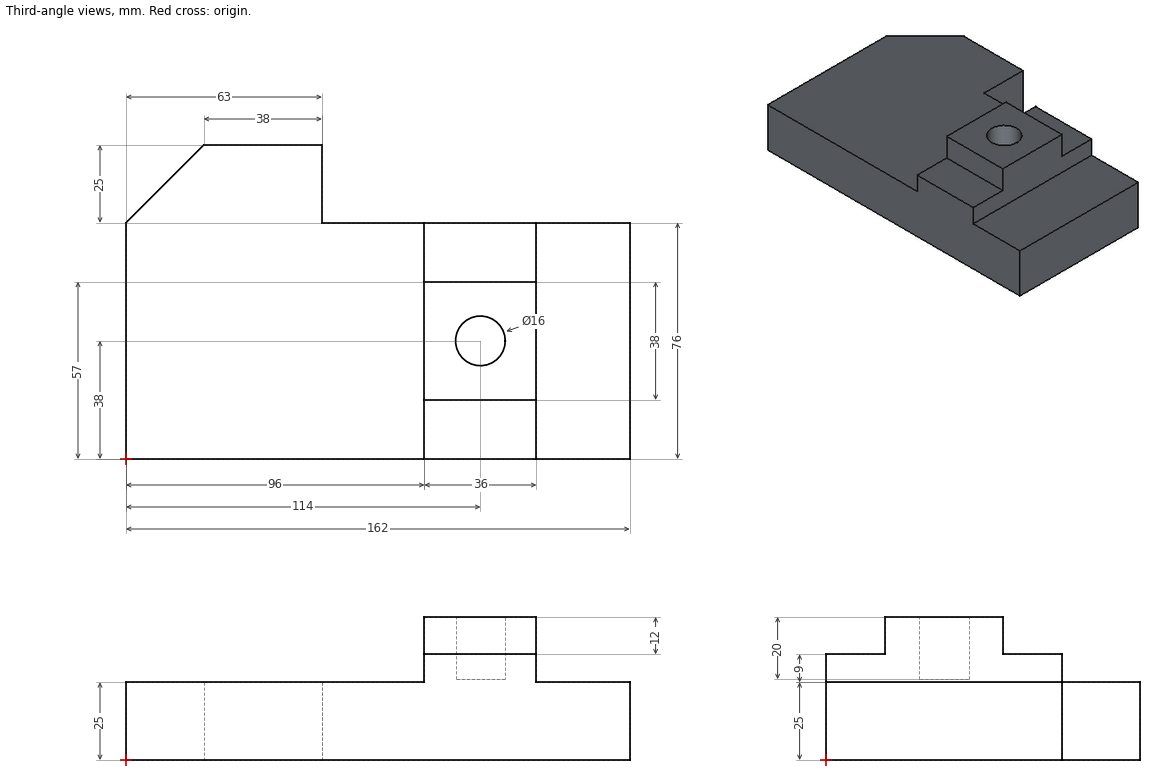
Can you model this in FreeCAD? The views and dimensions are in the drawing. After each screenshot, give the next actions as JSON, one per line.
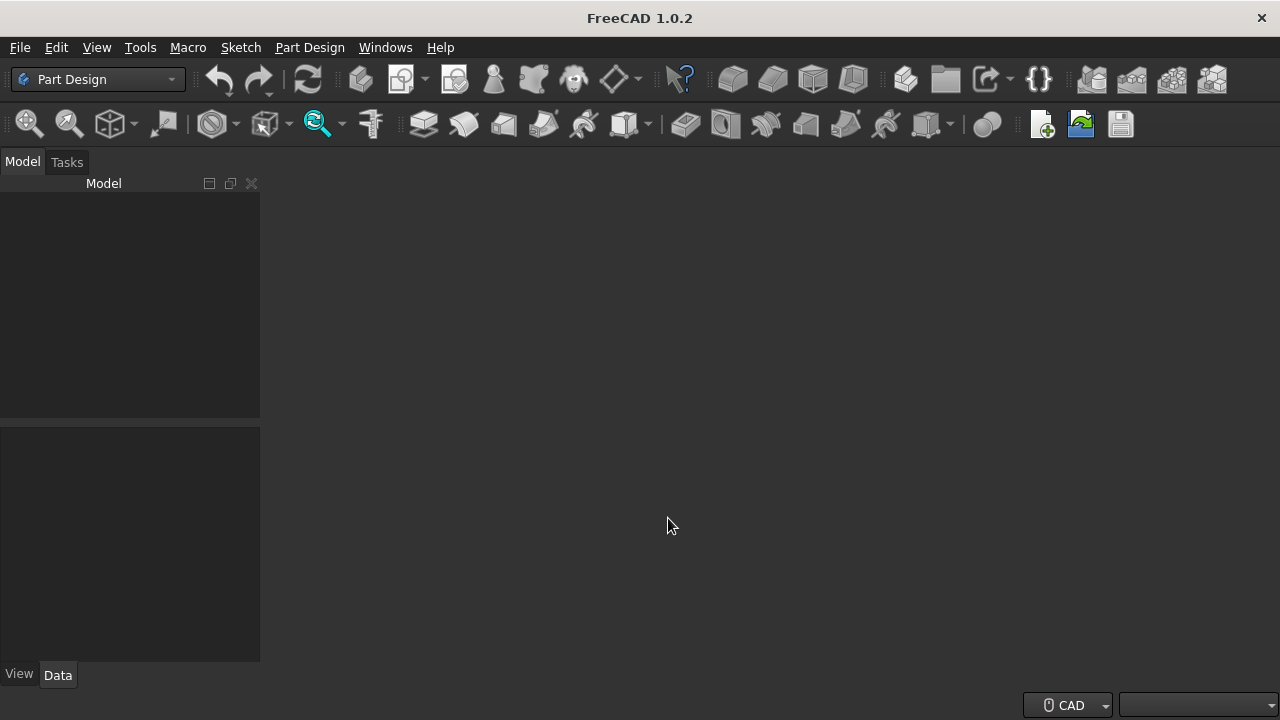
{"action": "key", "text": "ctrl+n"}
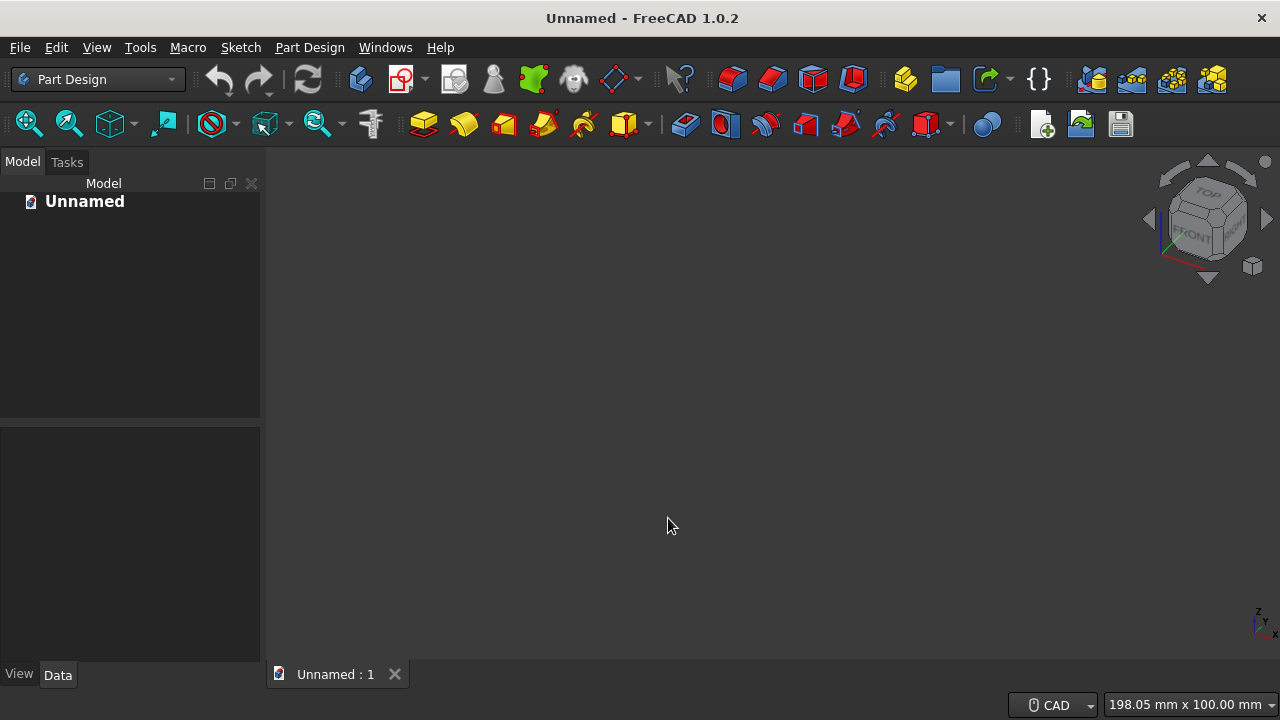
{"action": "left_click", "coordinate": [402, 80]}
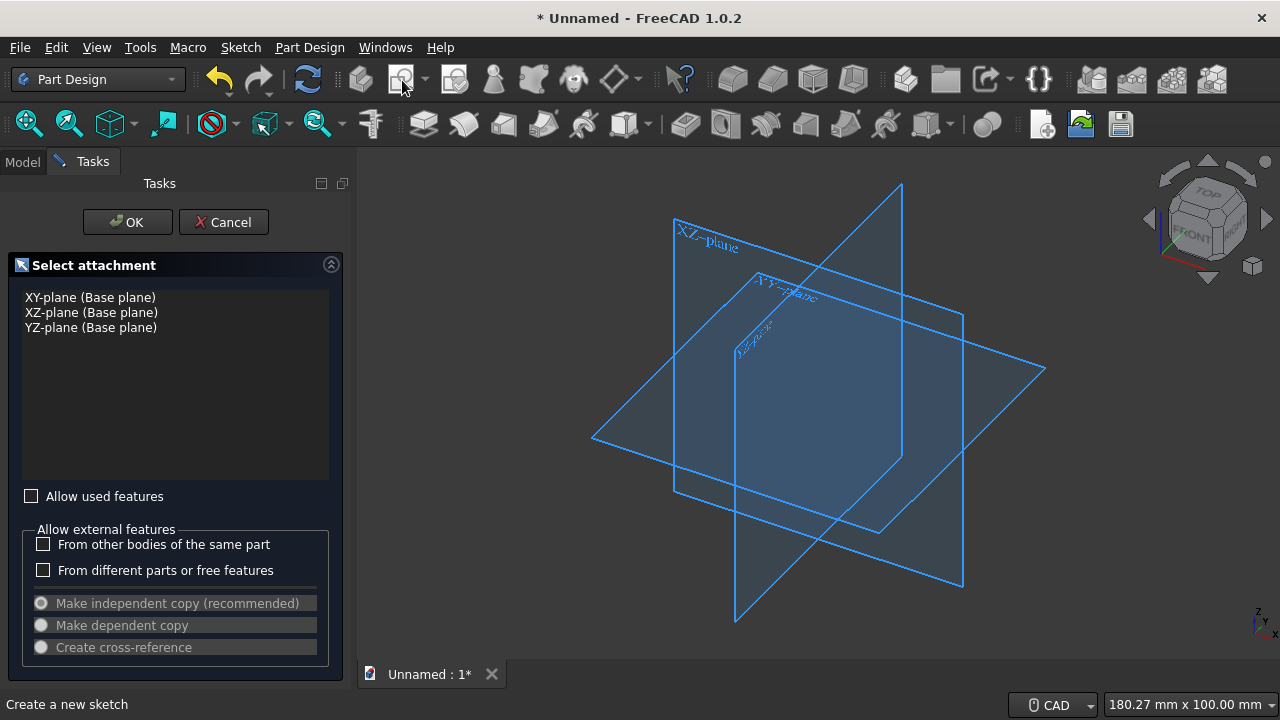
{"action": "left_click", "coordinate": [82, 298]}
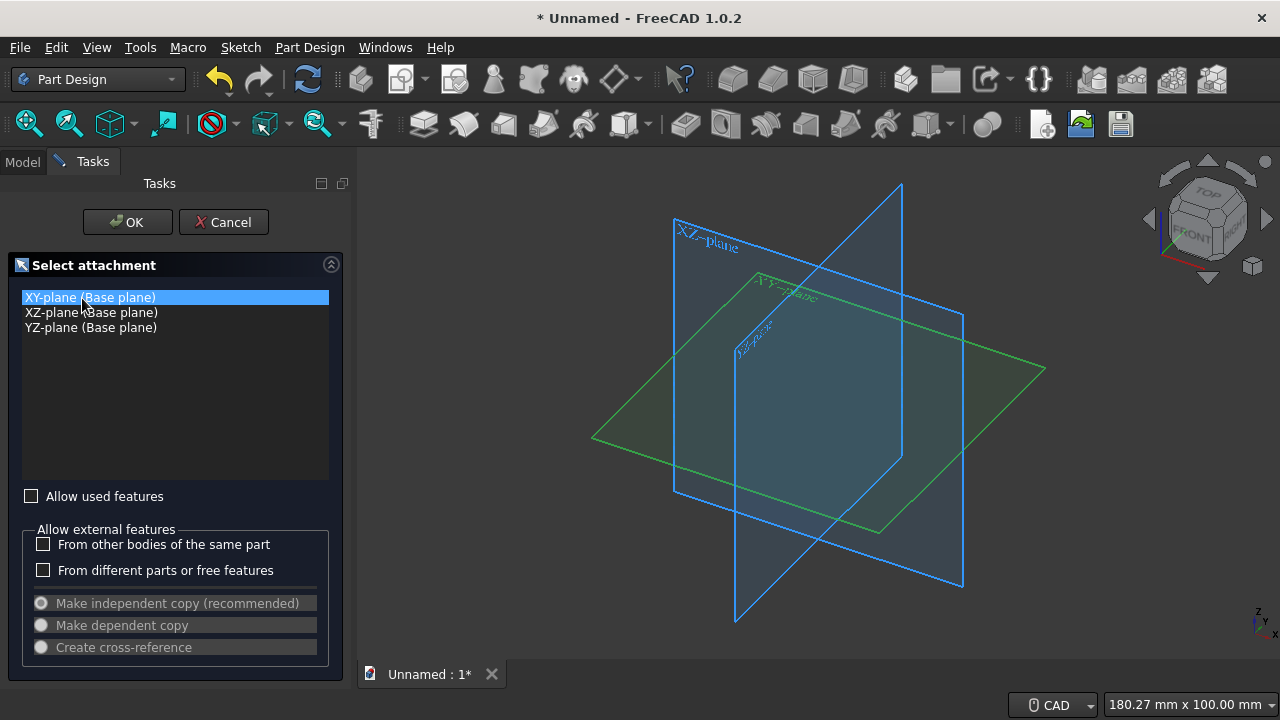
{"action": "left_click", "coordinate": [128, 222]}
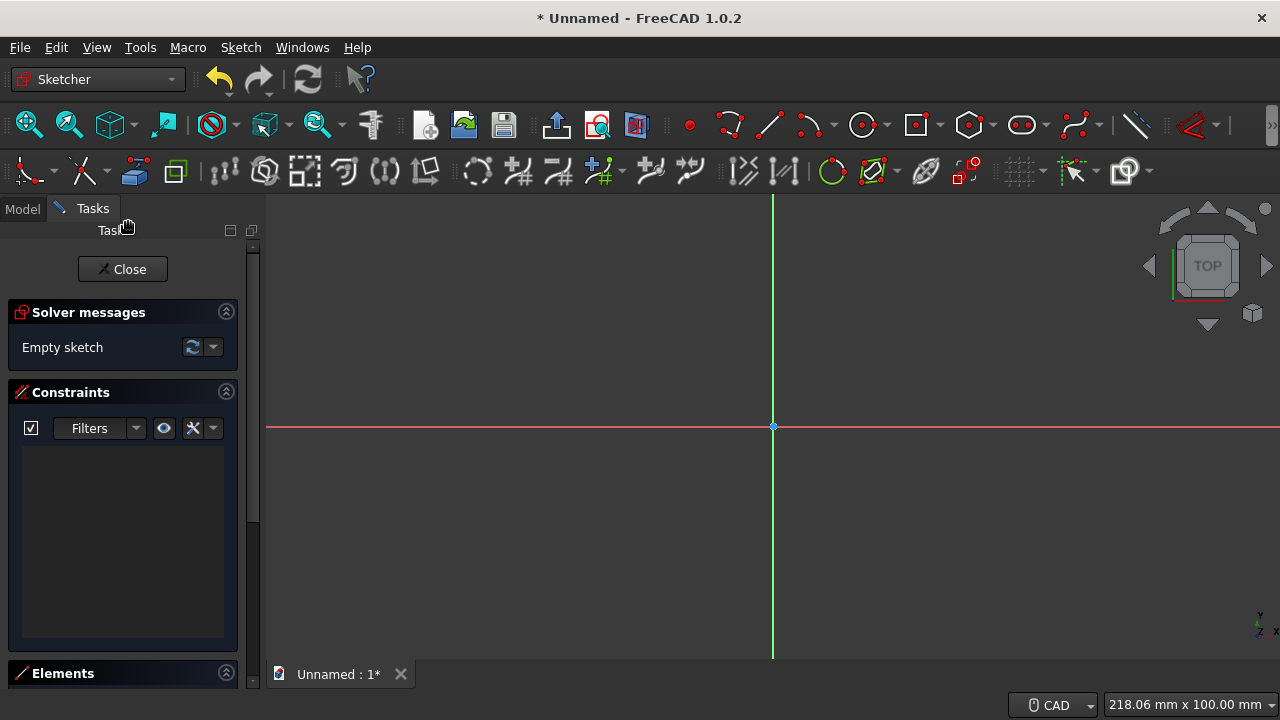
{"action": "scroll", "coordinate": [294, 631], "scroll_direction": "down", "scroll_amount": 3}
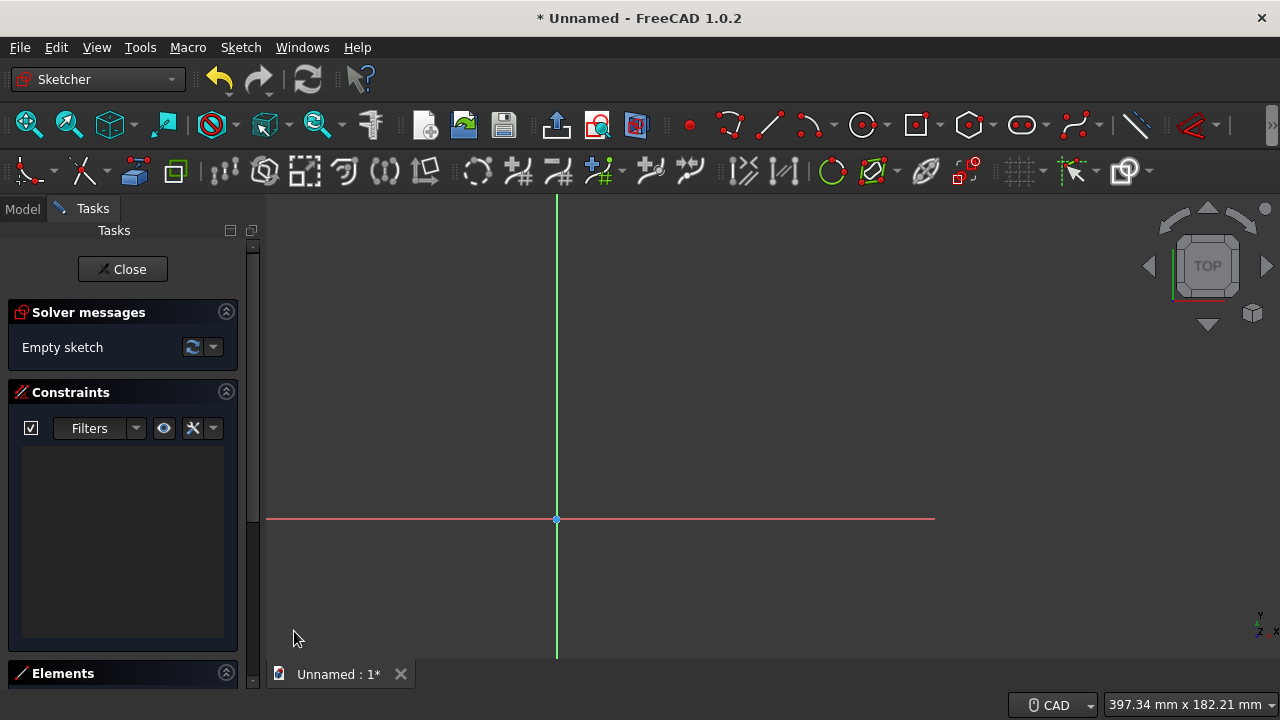
{"action": "scroll", "coordinate": [884, 414], "scroll_direction": "up", "scroll_amount": 2}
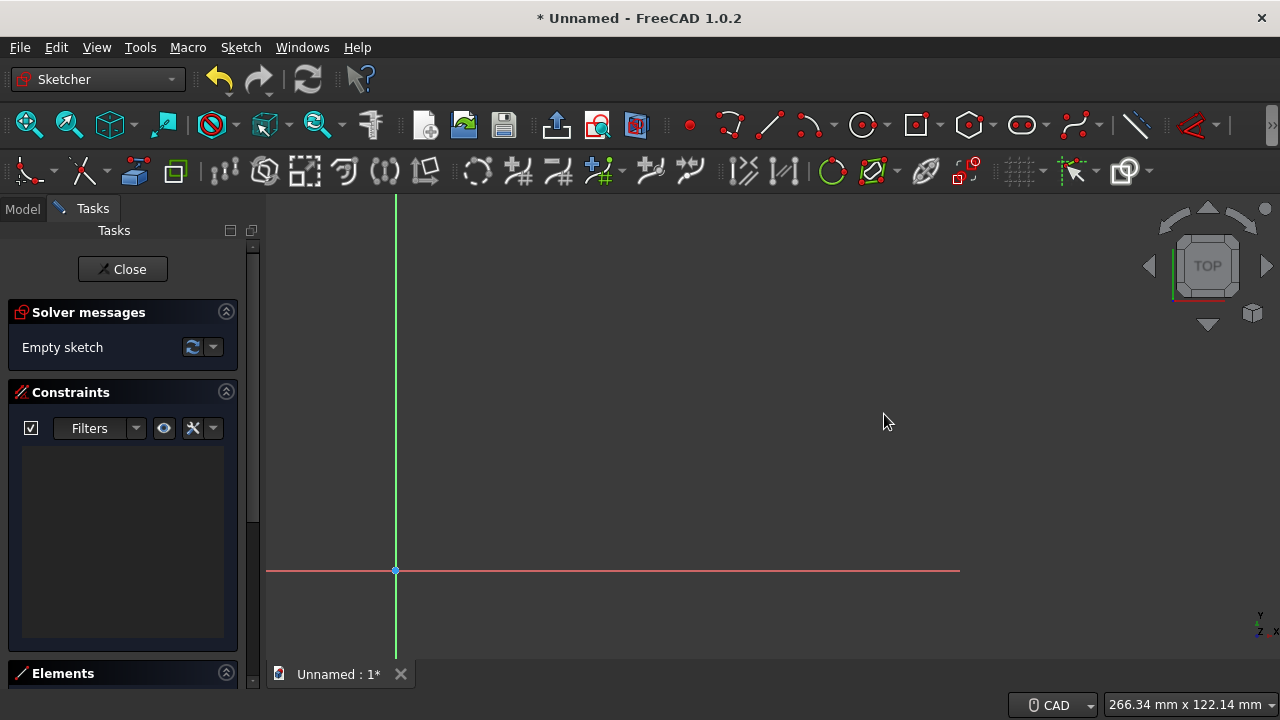
{"action": "key", "text": "g r"}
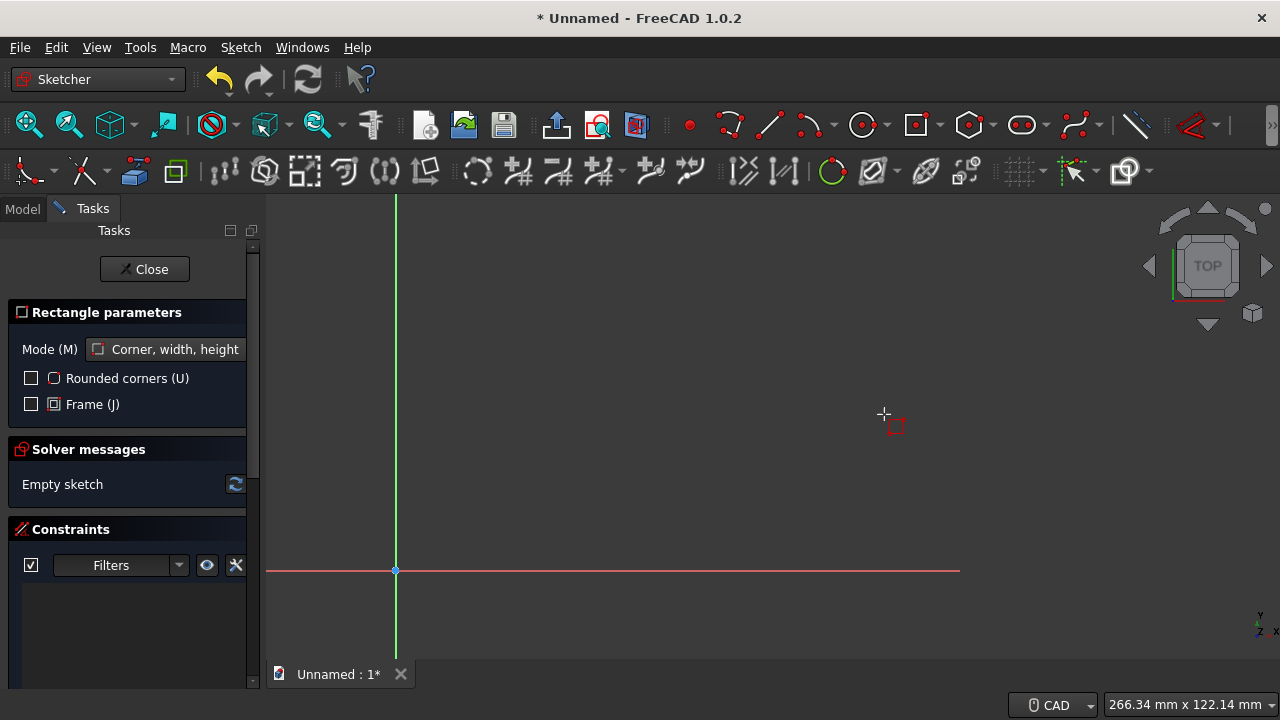
{"action": "left_click", "coordinate": [396, 571]}
{"action": "left_click", "coordinate": [1012, 281]}
{"action": "key", "text": "Escape"}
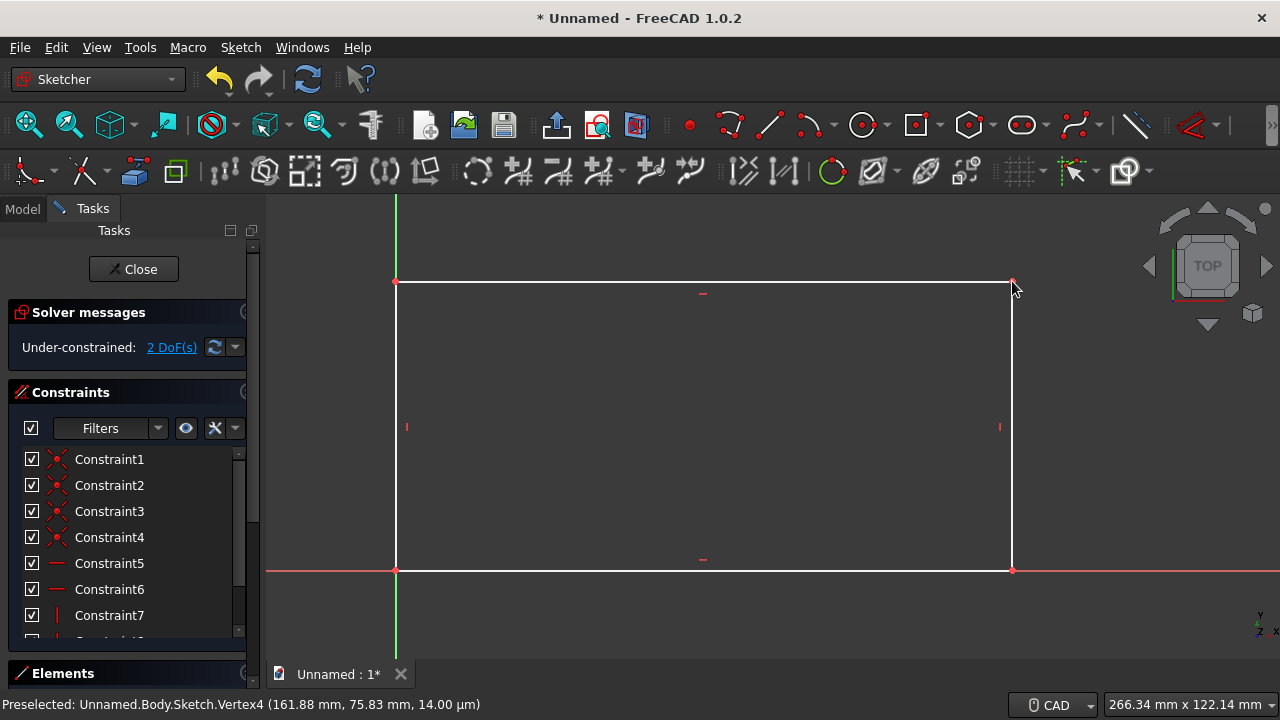
{"action": "left_click", "coordinate": [1012, 484]}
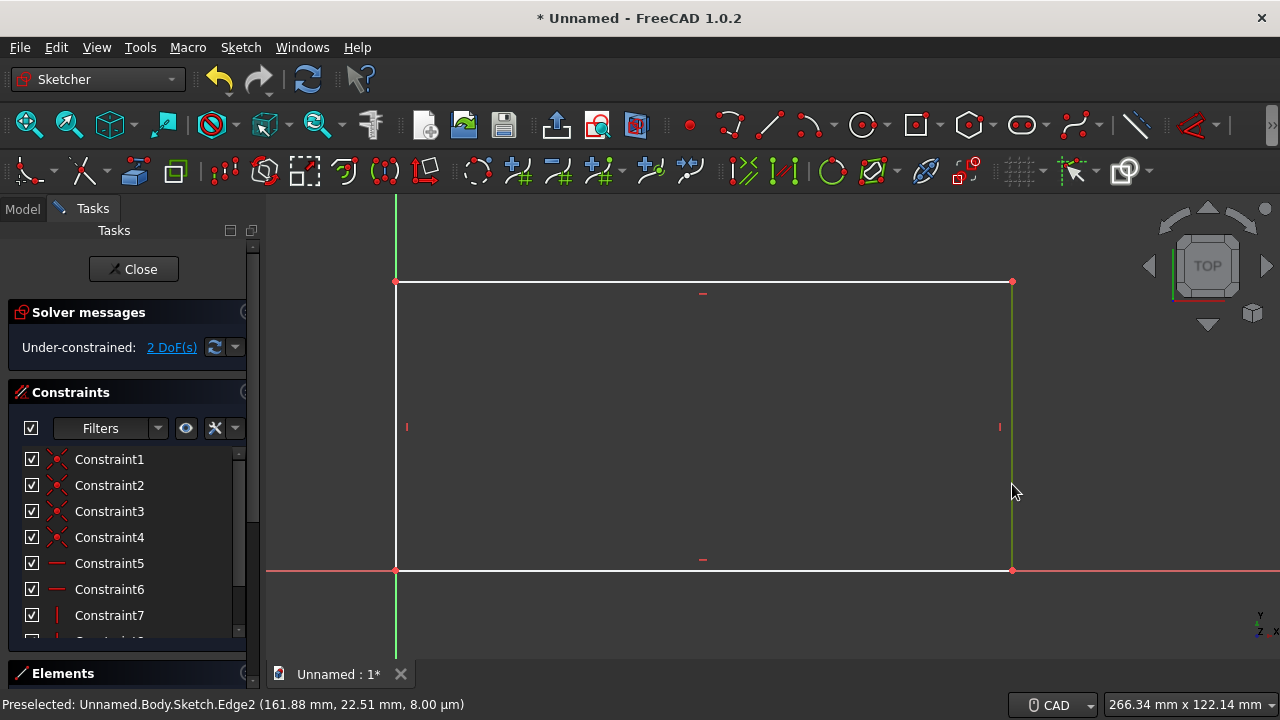
{"action": "key", "text": "i"}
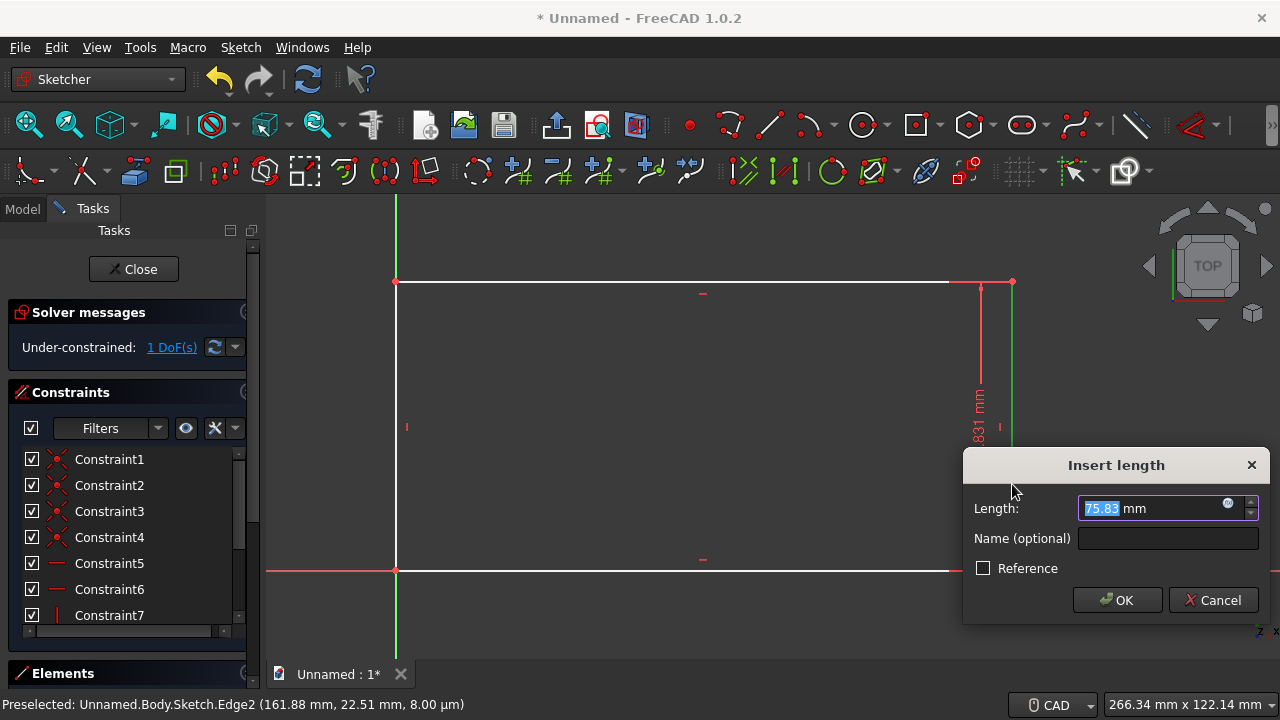
{"action": "type", "text": "76"}
{"action": "key", "text": "Return"}